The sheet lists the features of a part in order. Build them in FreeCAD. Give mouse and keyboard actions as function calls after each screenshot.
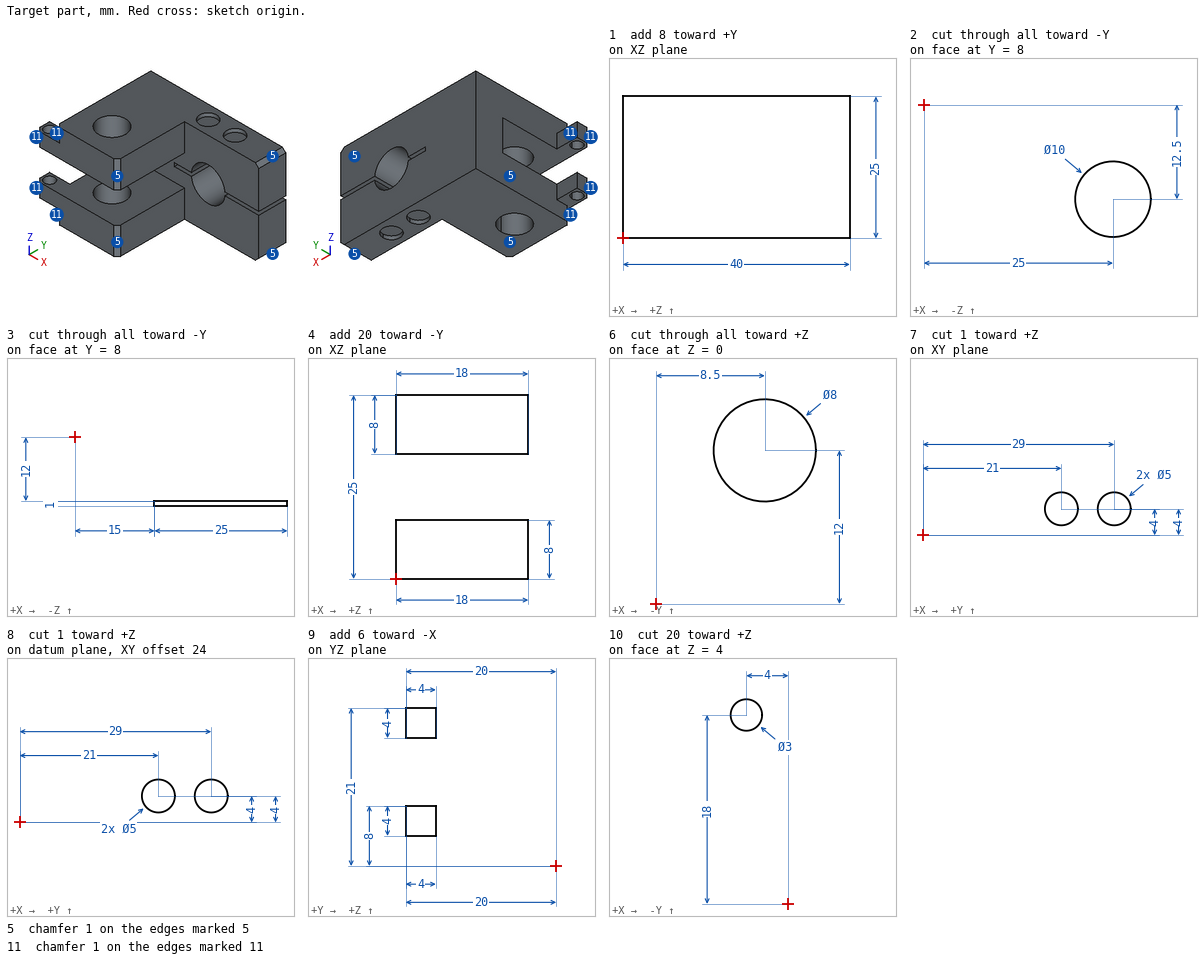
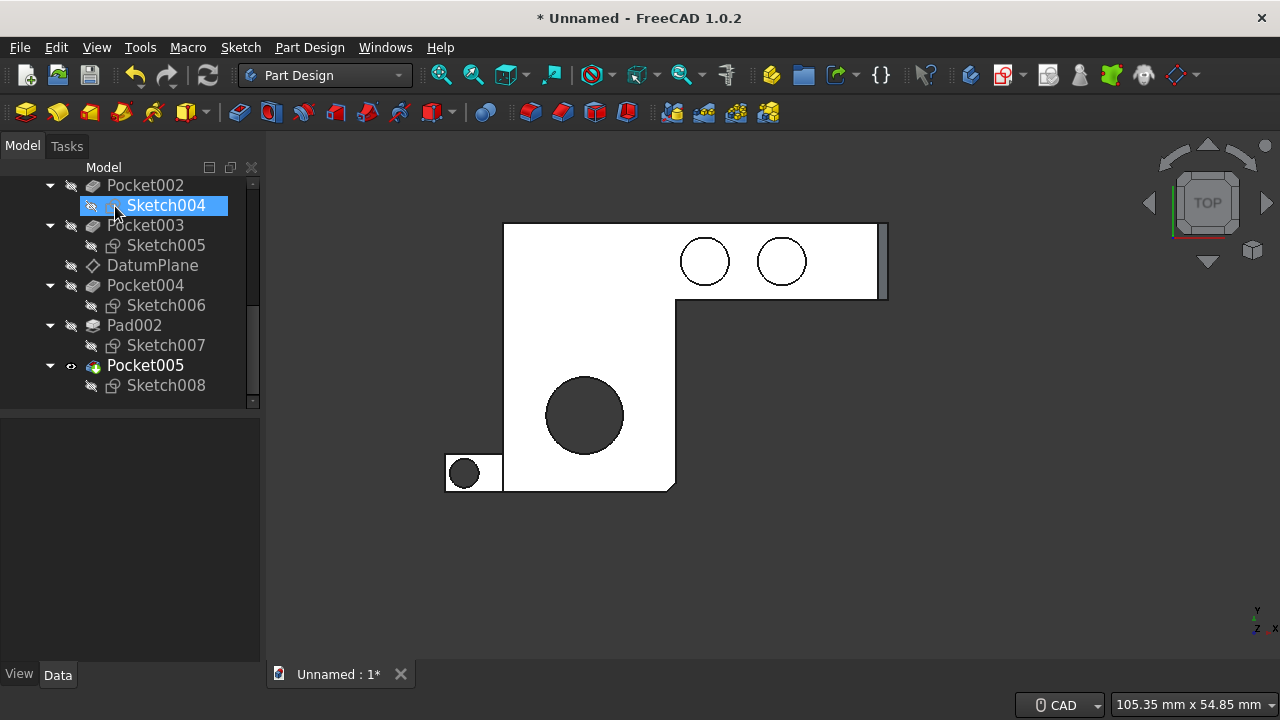
key(1)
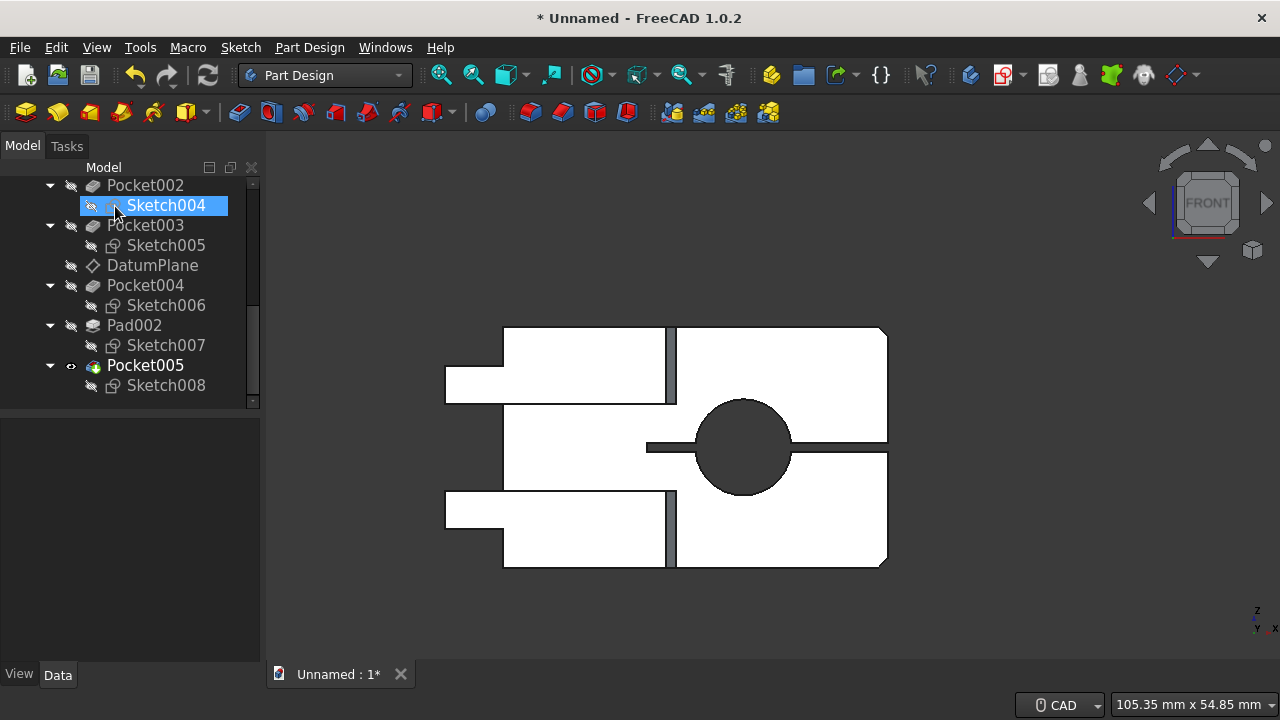
click(503, 547)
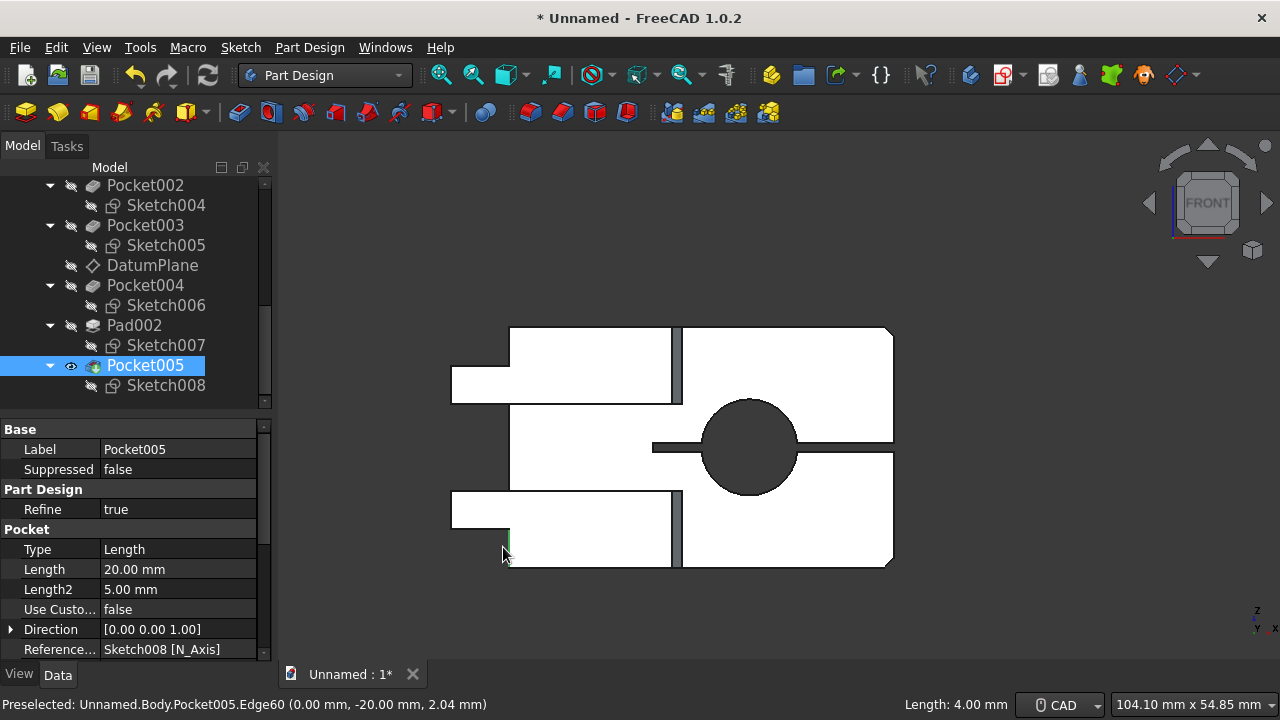
click(451, 509, ctrl)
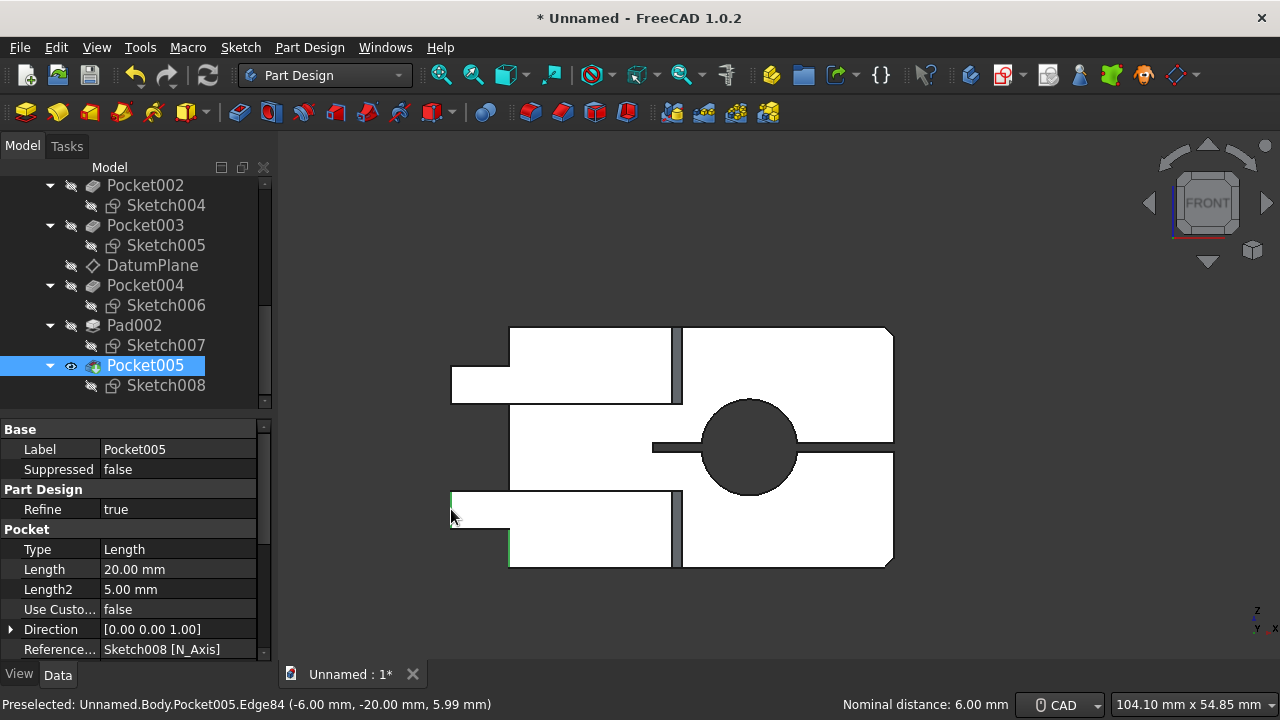
click(451, 384, ctrl)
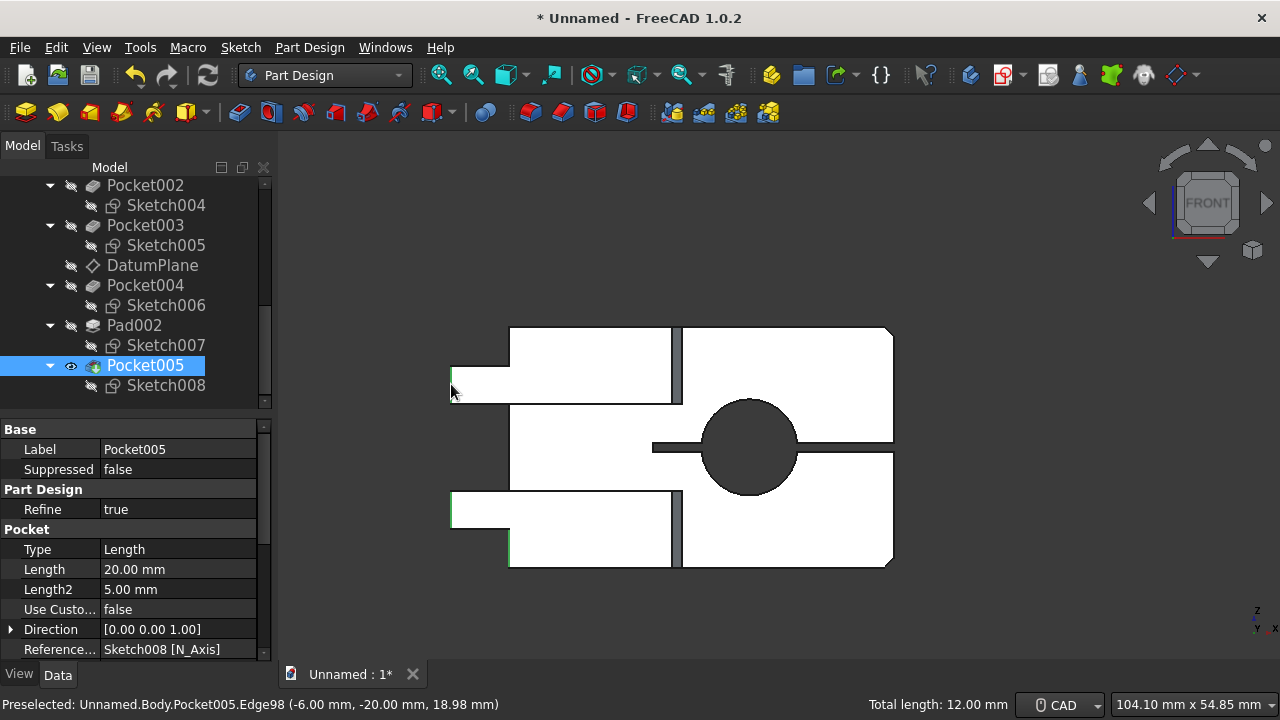
click(509, 345, ctrl)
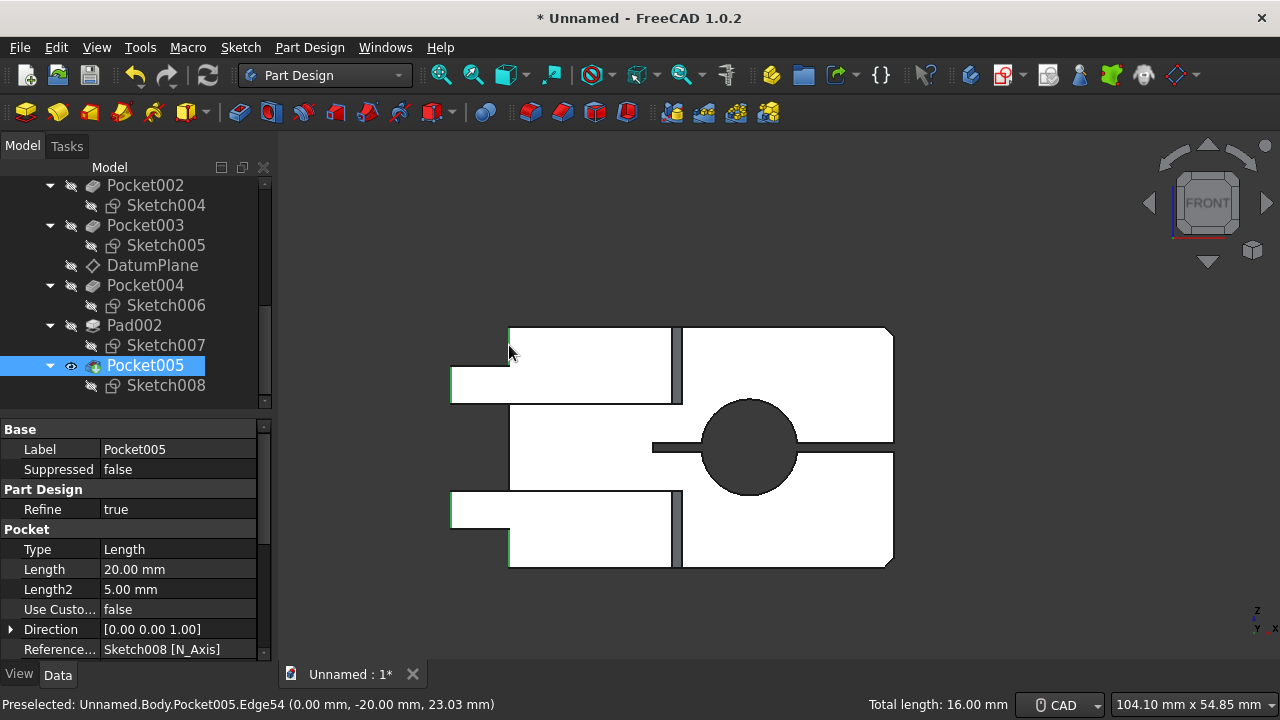
click(564, 112)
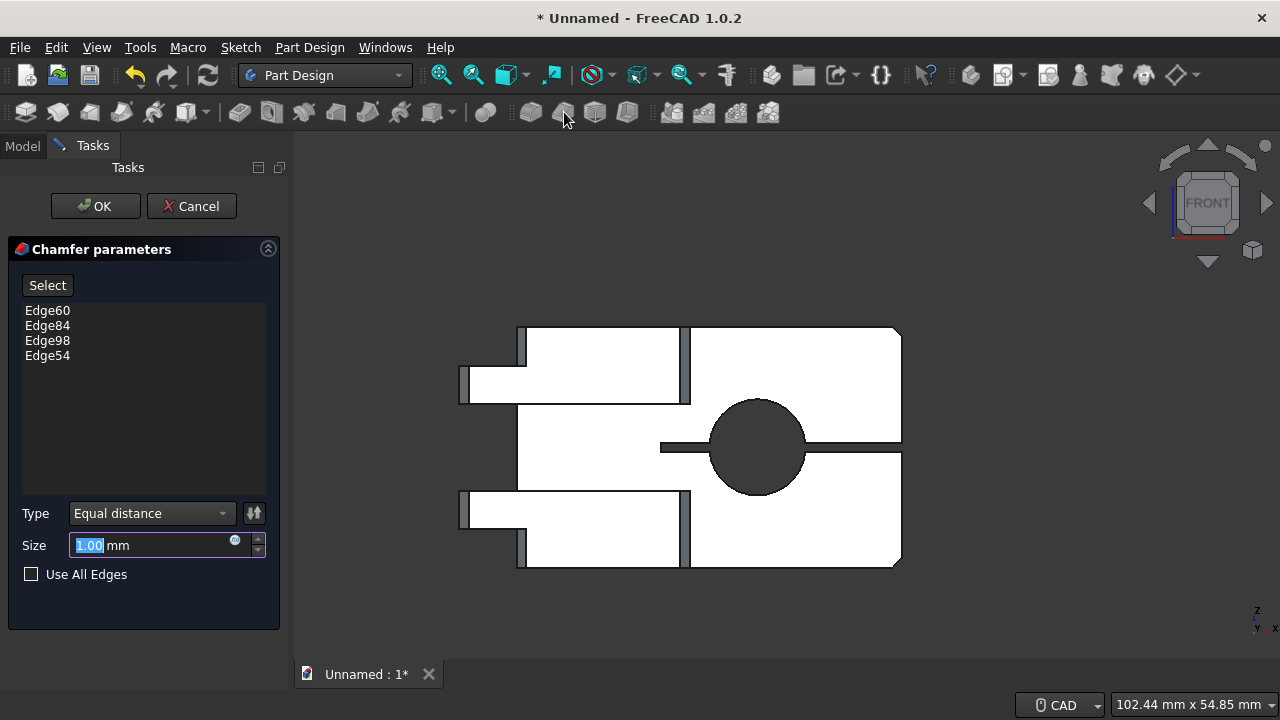
text(1)
key(Tab)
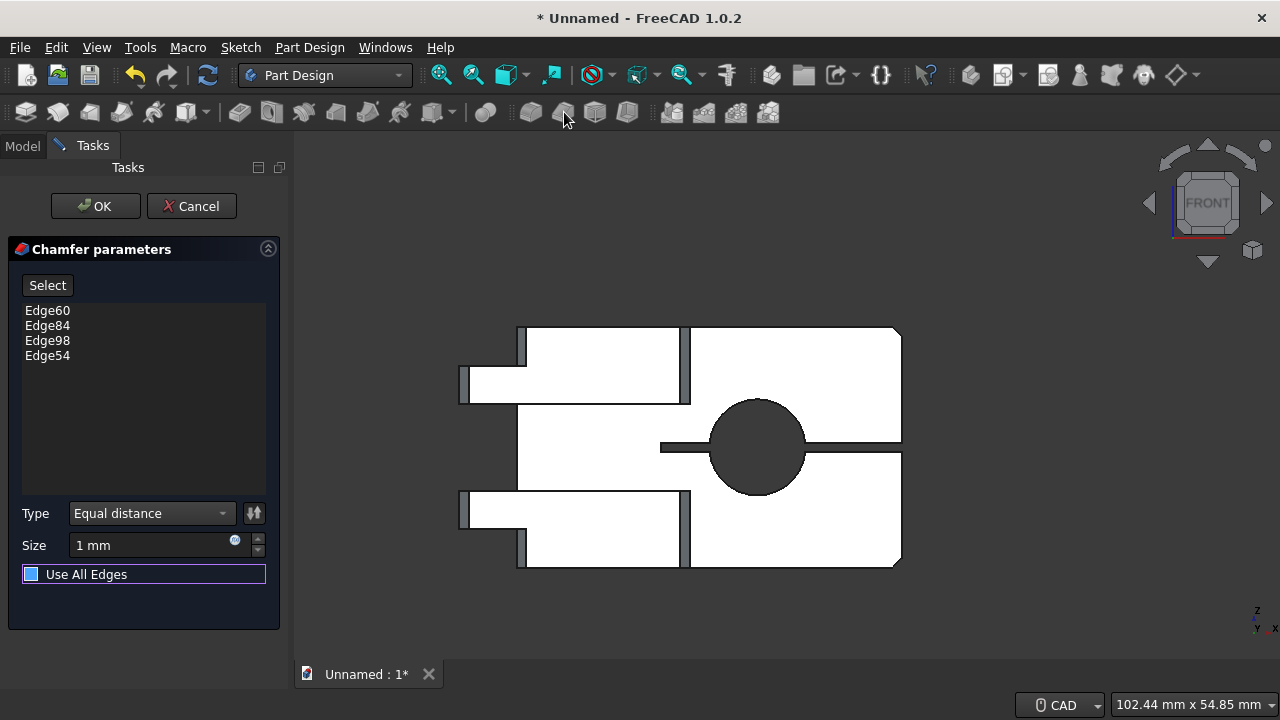
click(96, 206)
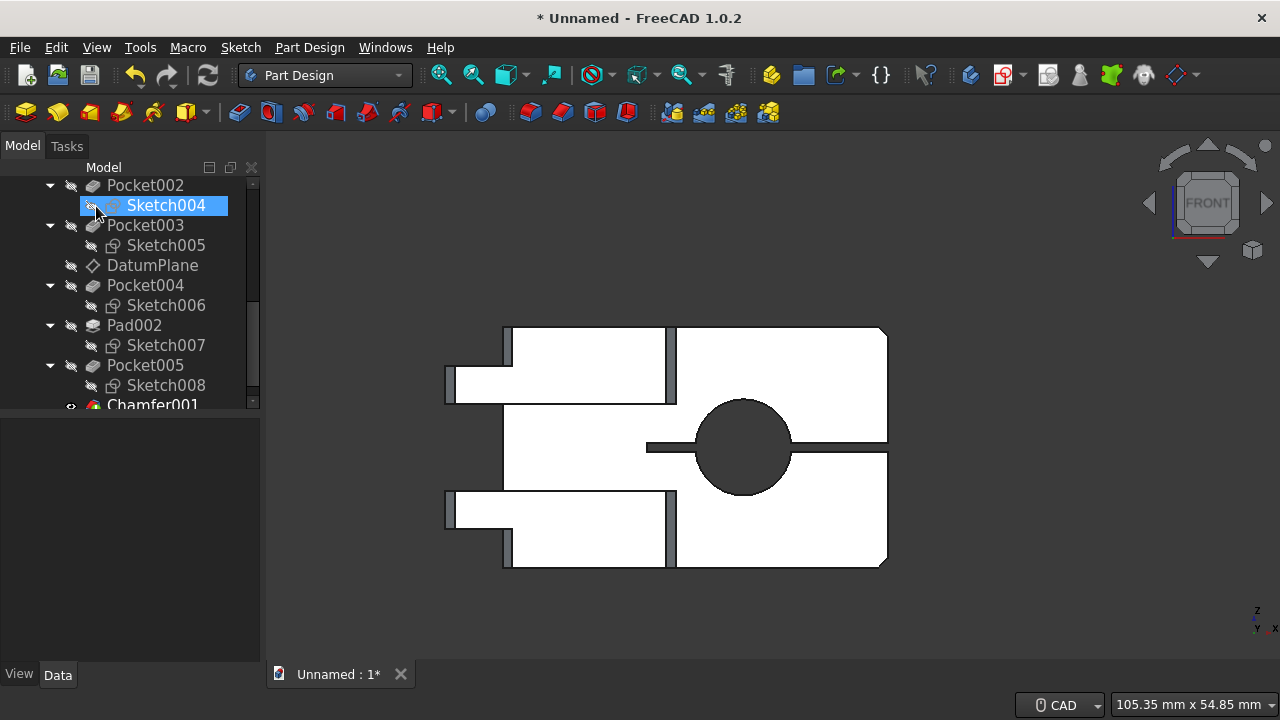
key(0)